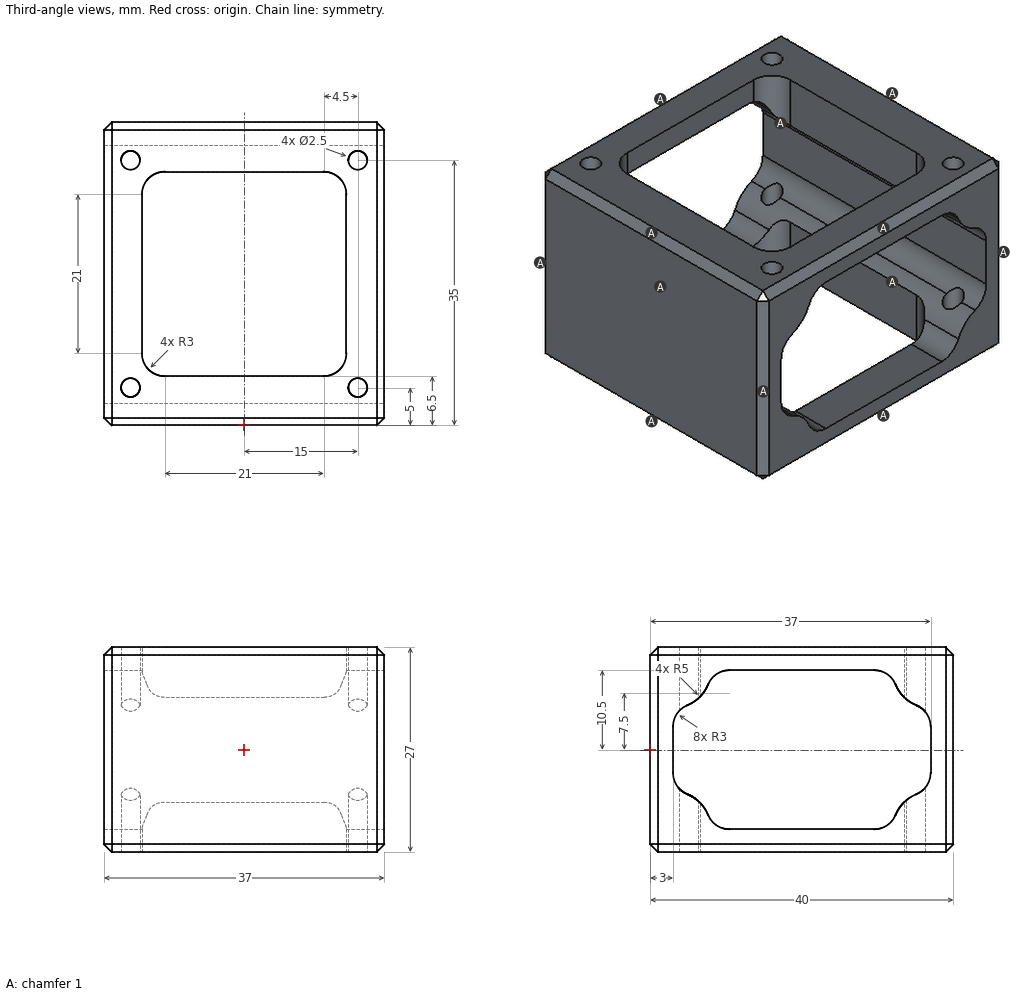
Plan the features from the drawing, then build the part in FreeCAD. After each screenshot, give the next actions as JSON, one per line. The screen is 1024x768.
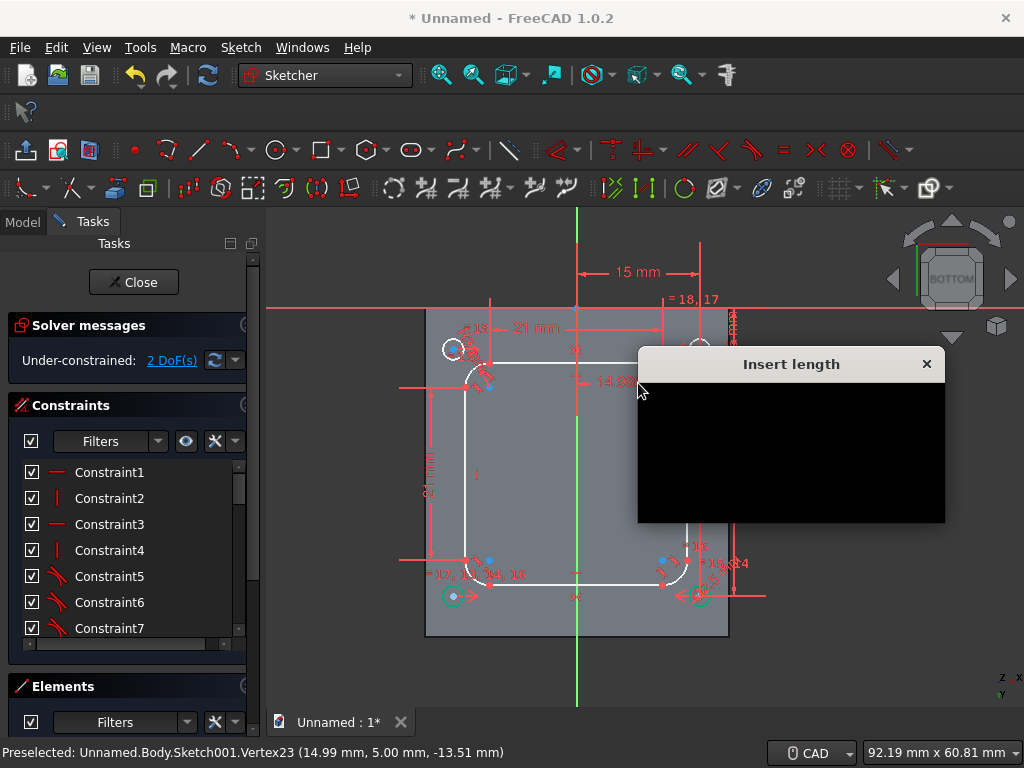
{"action": "type", "text": "15"}
{"action": "key", "text": "Return"}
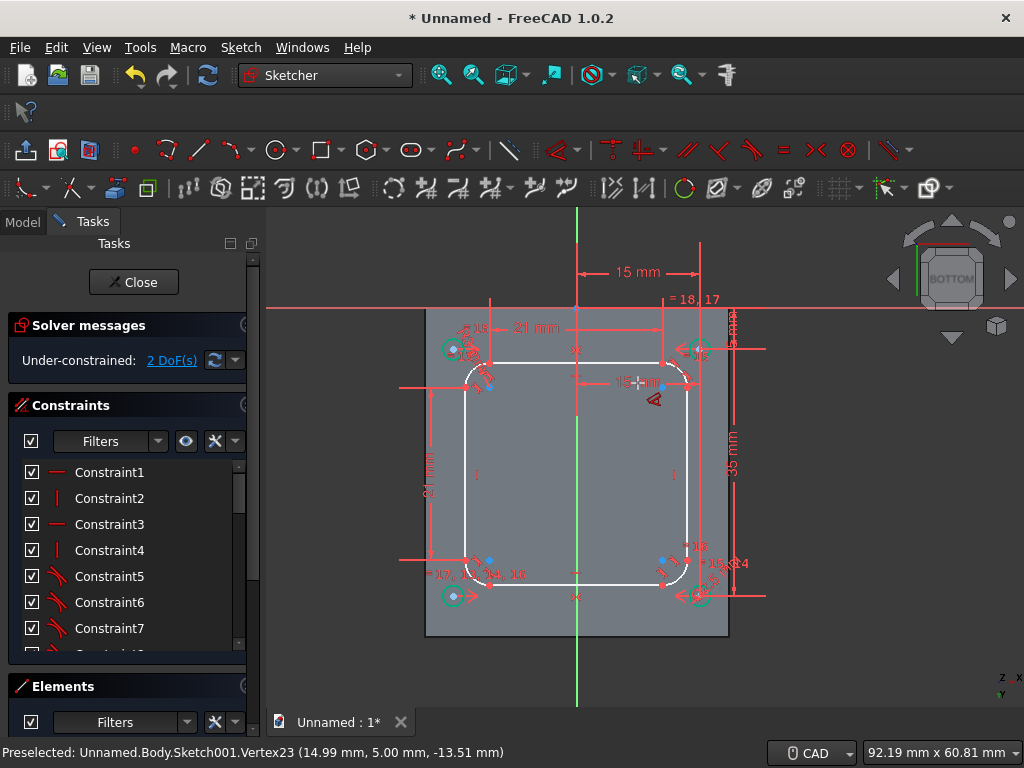
{"action": "left_click", "coordinate": [663, 363]}
{"action": "left_click", "coordinate": [745, 355]}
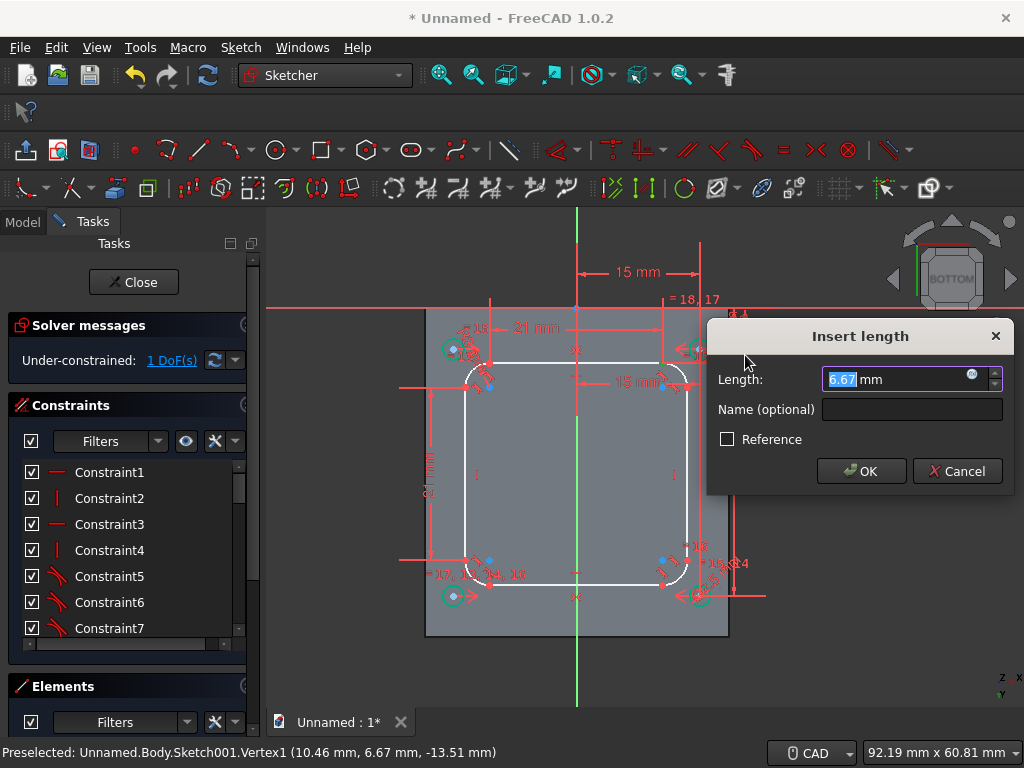
{"action": "type", "text": "6.5"}
{"action": "key", "text": "Return"}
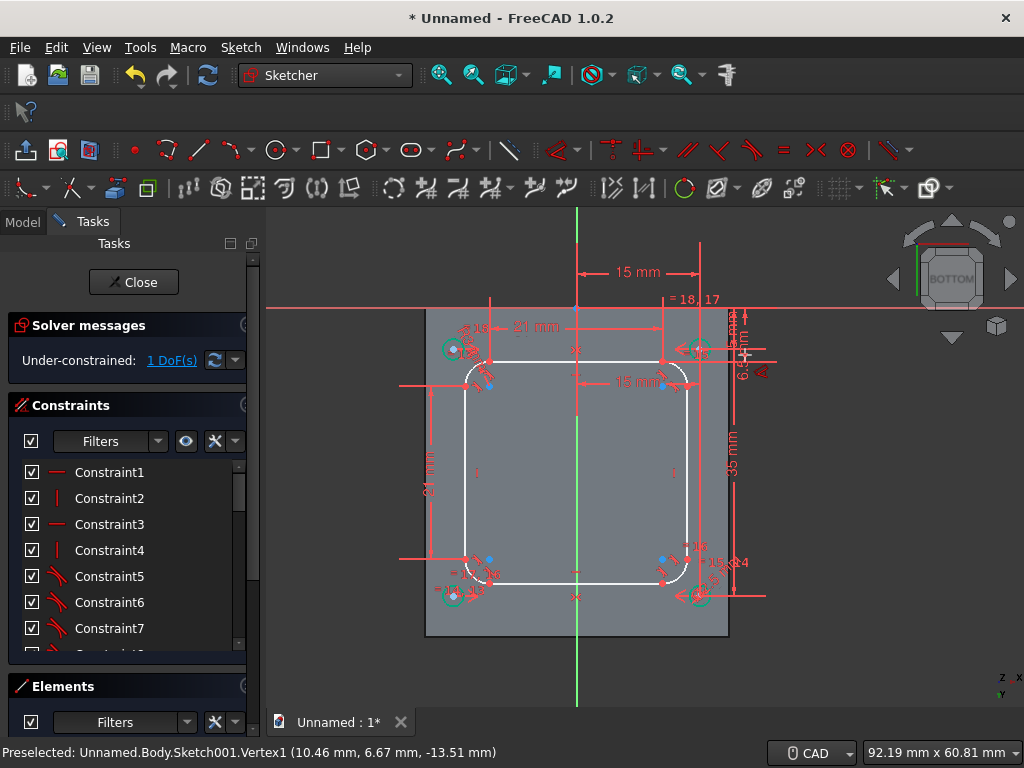
{"action": "left_click", "coordinate": [663, 584]}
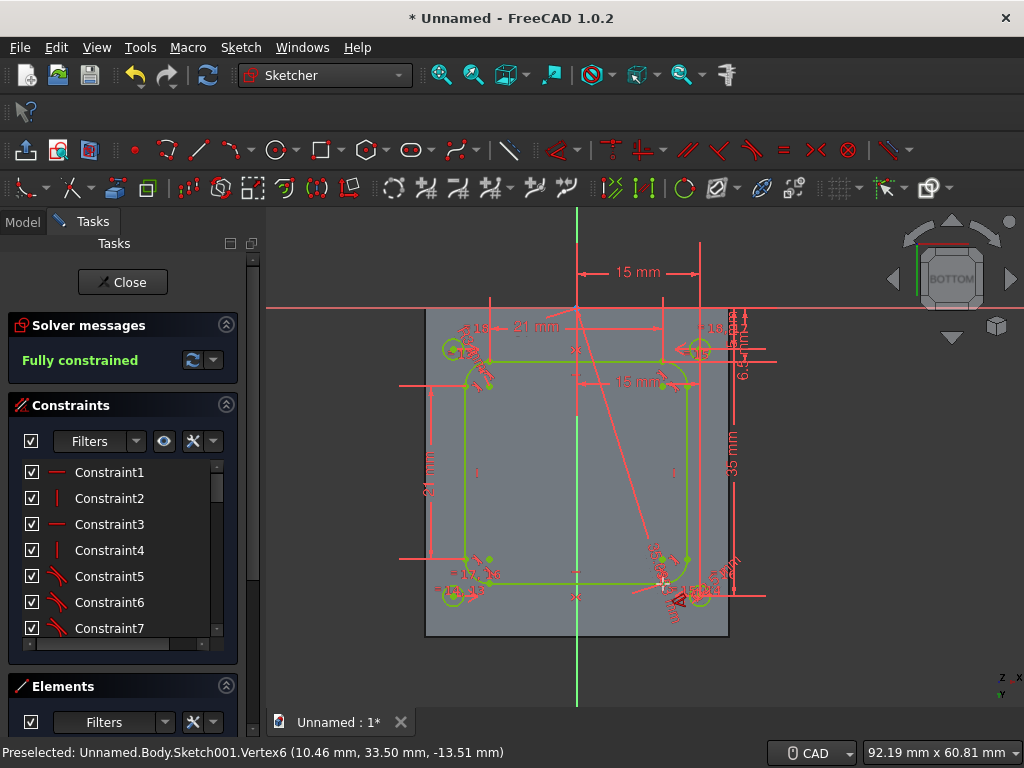
{"action": "left_click", "coordinate": [700, 596]}
{"action": "left_click", "coordinate": [681, 630]}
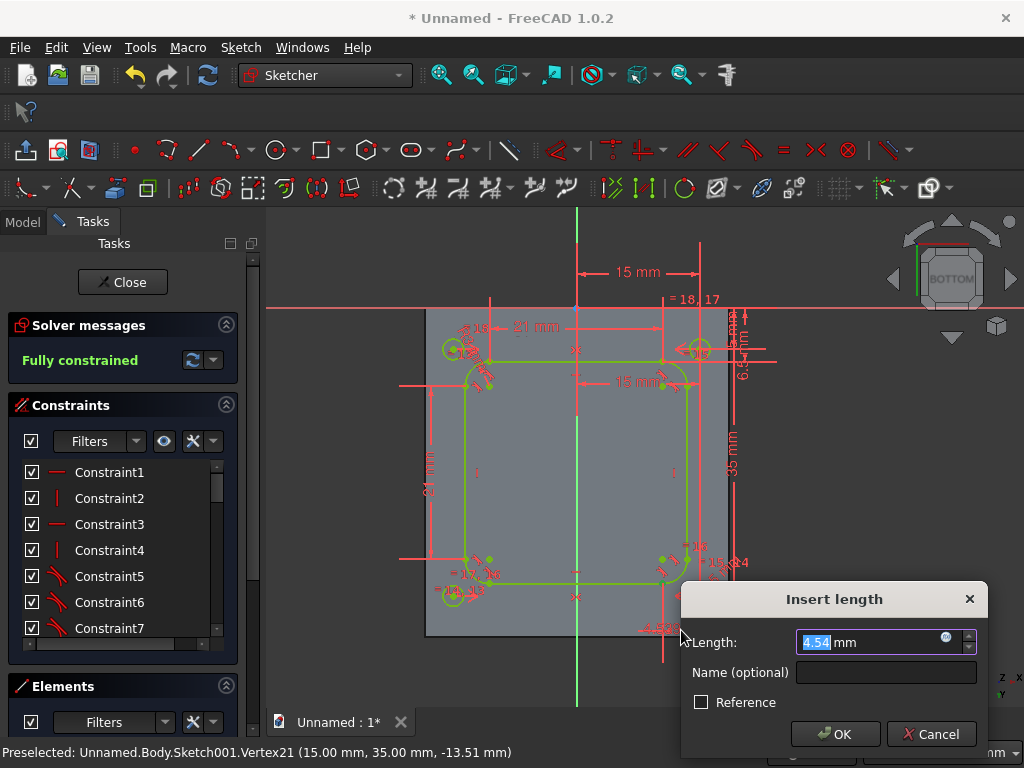
{"action": "type", "text": "4.5"}
{"action": "key", "text": "Return"}
{"action": "key", "text": "Escape"}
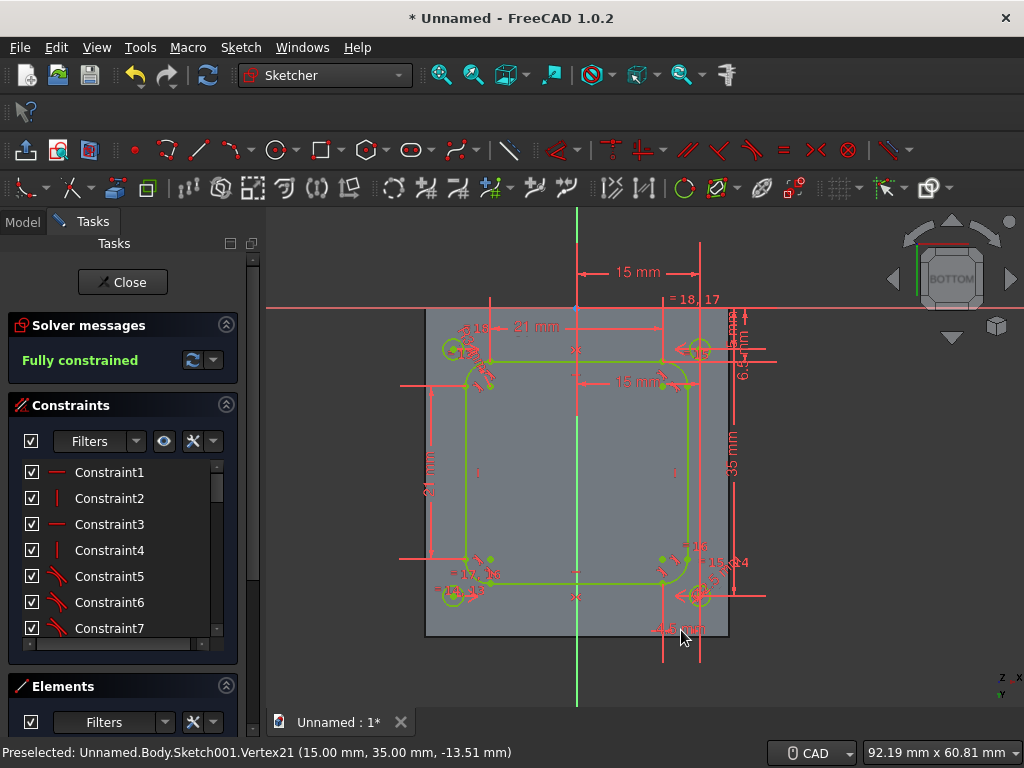
{"action": "left_click", "coordinate": [123, 282]}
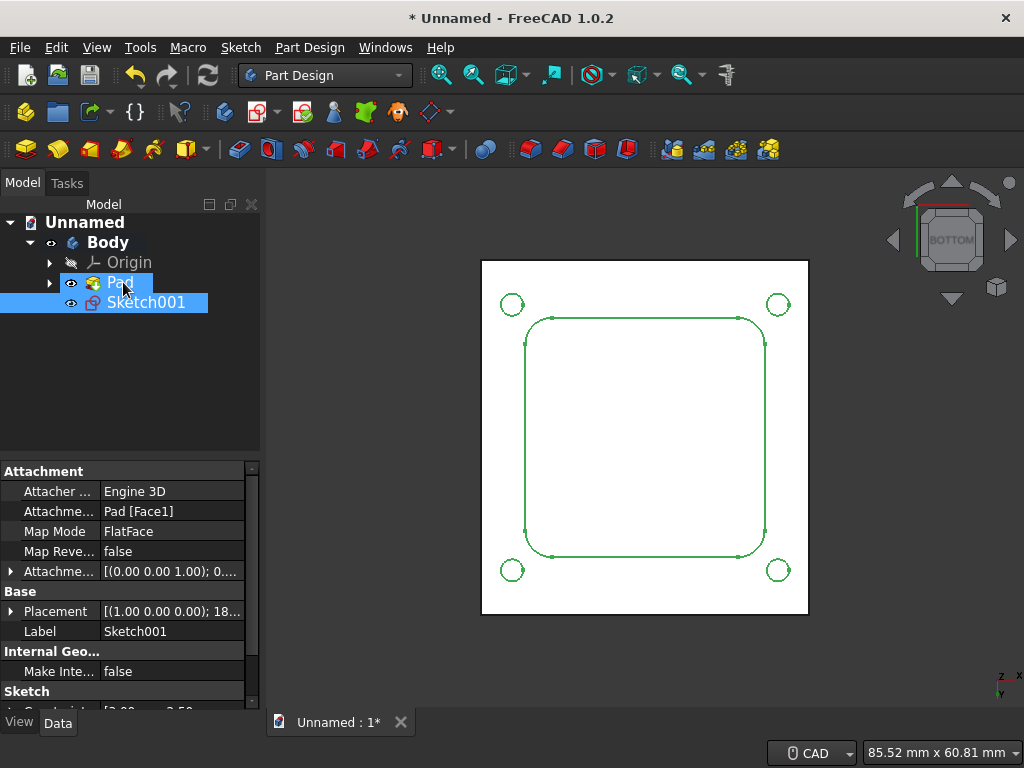
{"action": "left_click", "coordinate": [240, 150]}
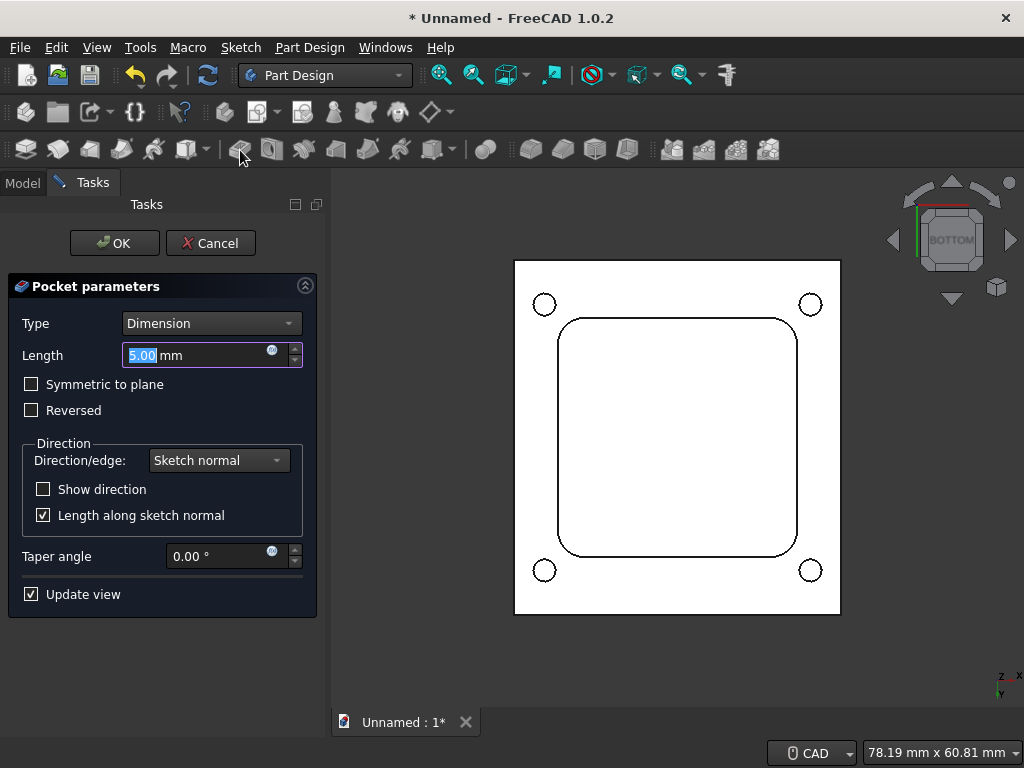
{"action": "left_click", "coordinate": [212, 324]}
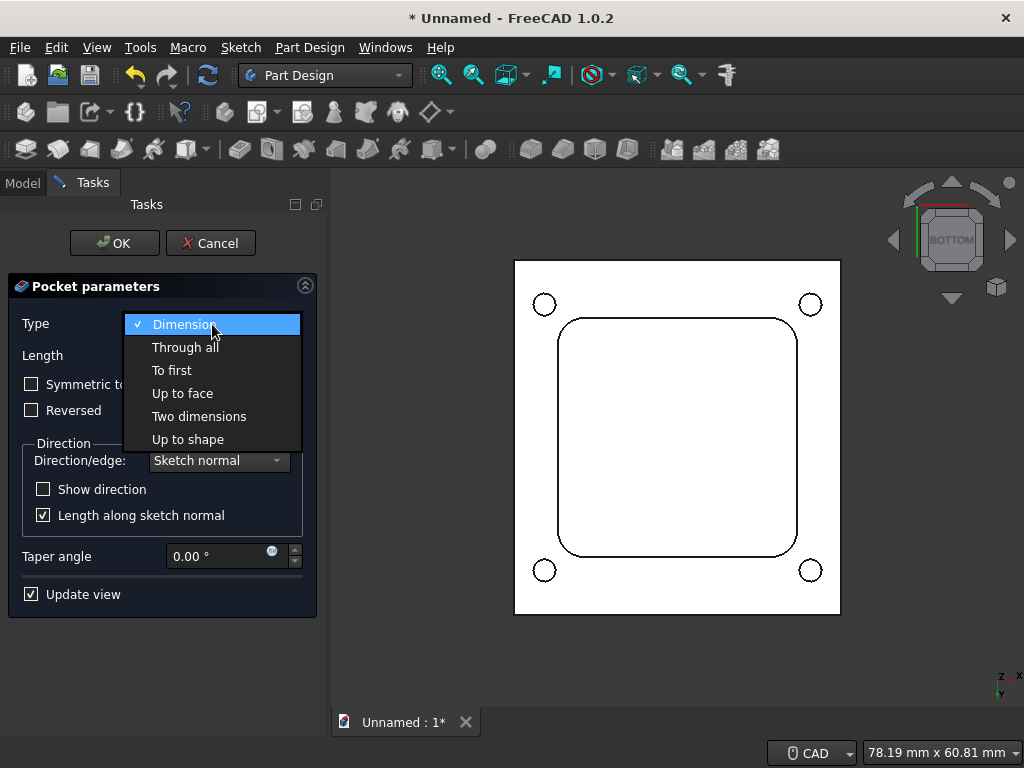
{"action": "left_click", "coordinate": [212, 348]}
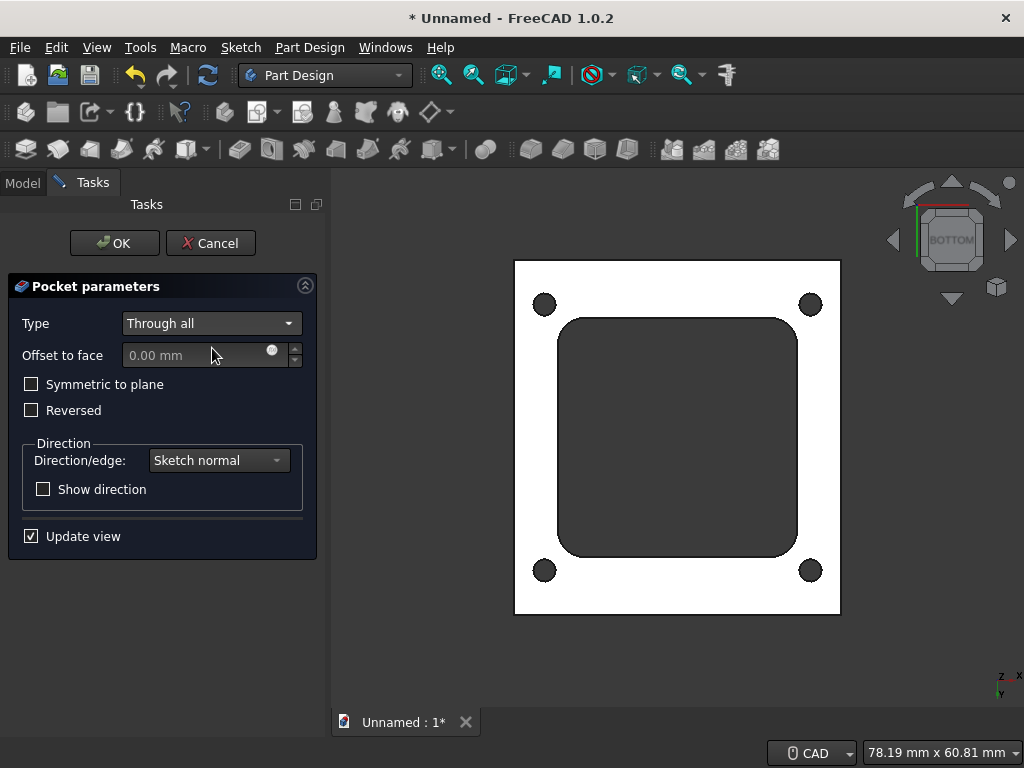
{"action": "left_click", "coordinate": [115, 243]}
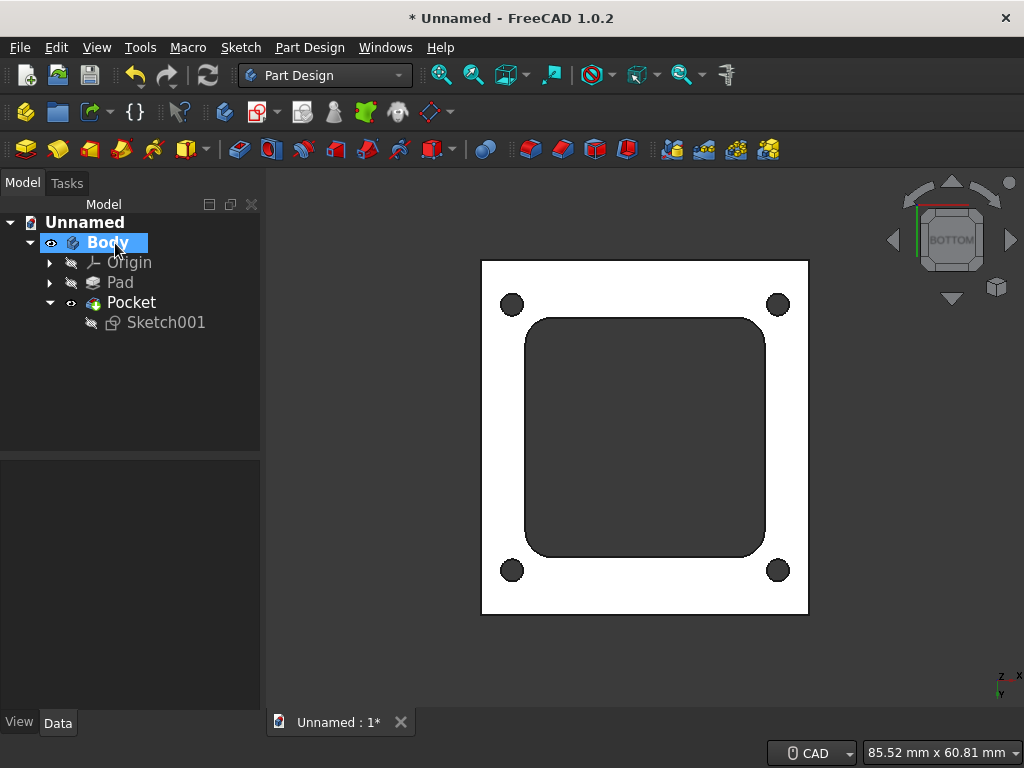
{"action": "key", "text": "6"}